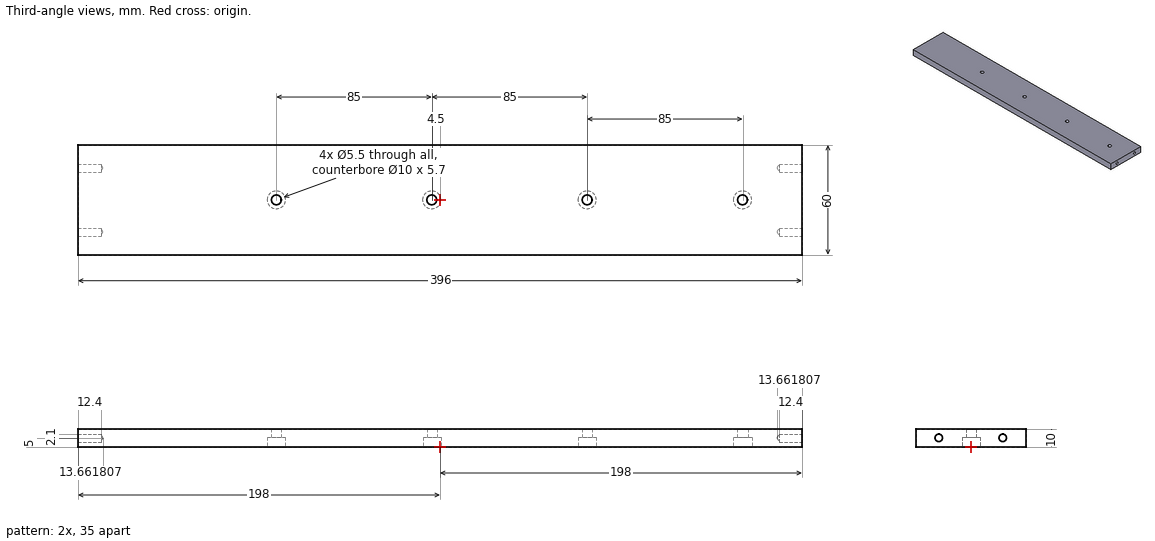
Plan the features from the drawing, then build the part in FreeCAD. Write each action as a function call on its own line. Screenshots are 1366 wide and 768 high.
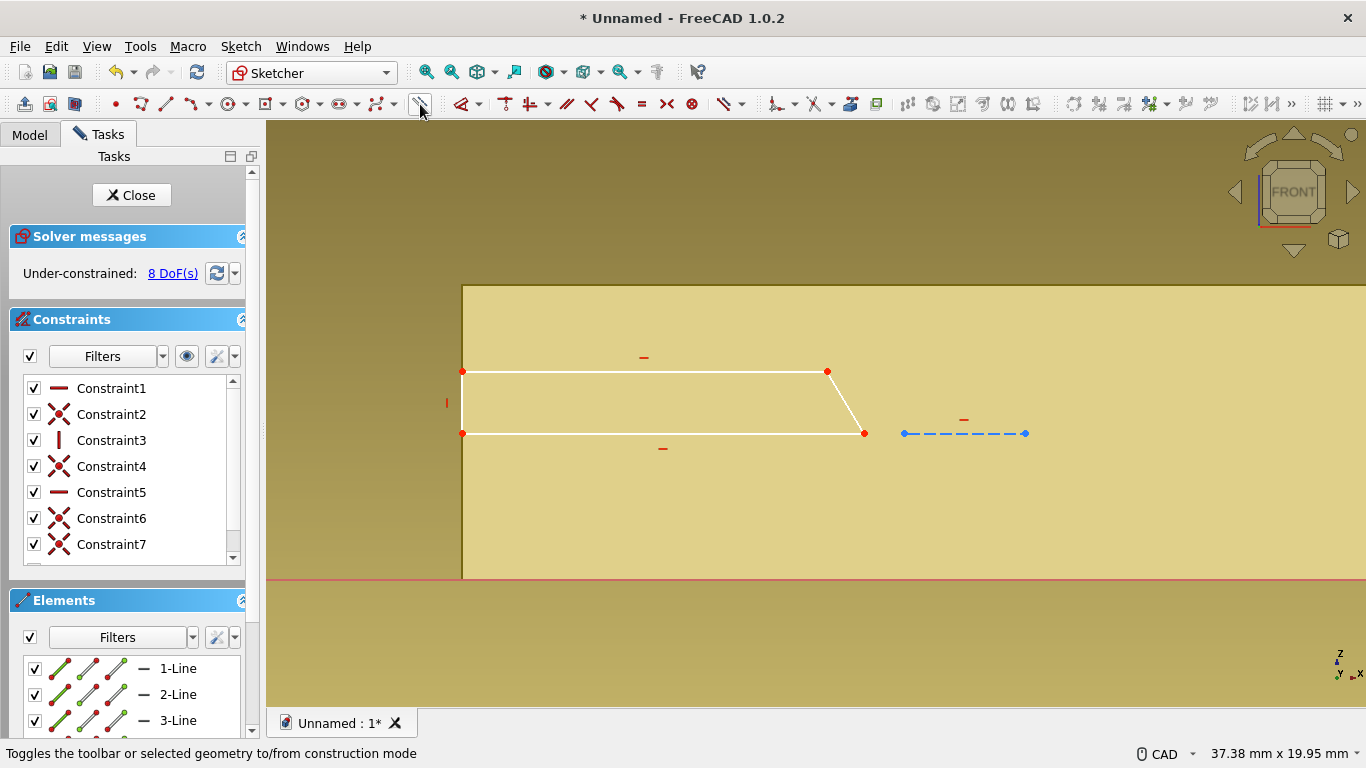
click(460, 104)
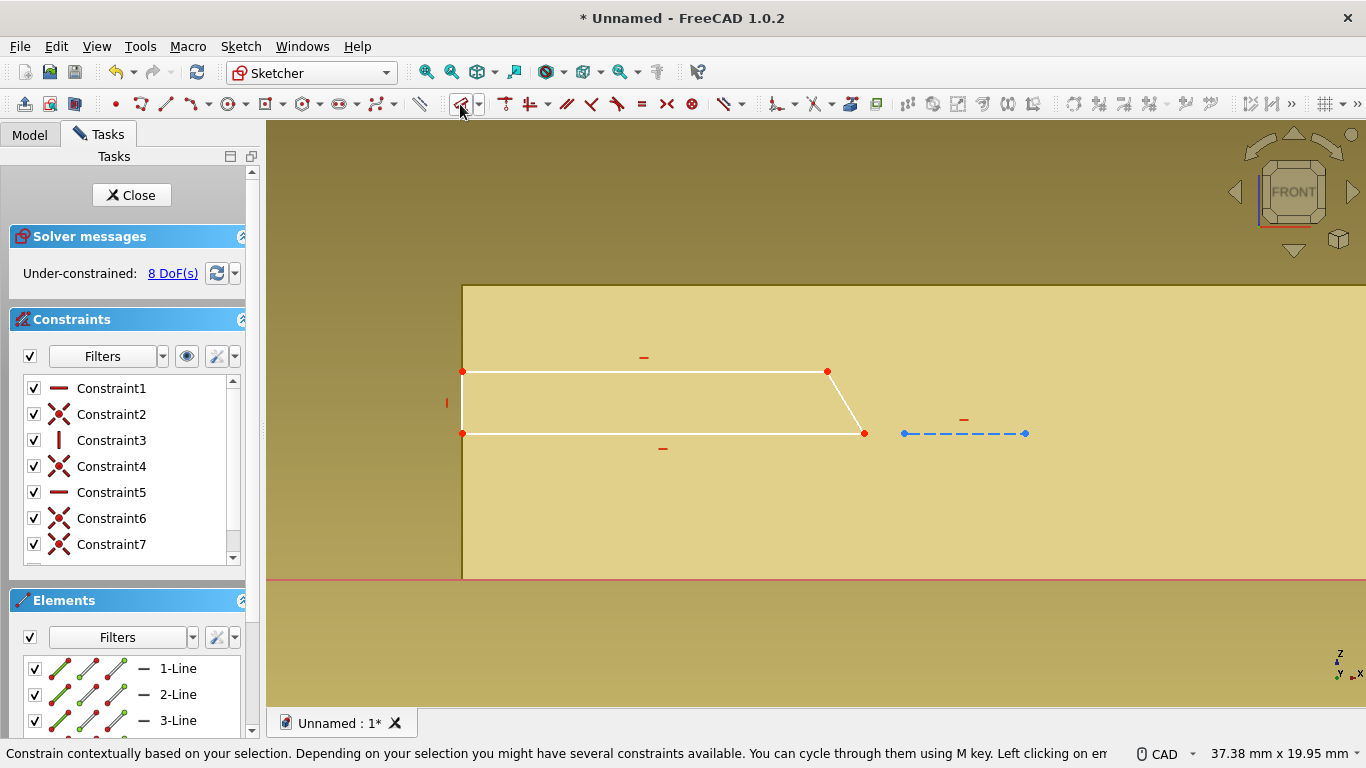
click(864, 434)
click(830, 507)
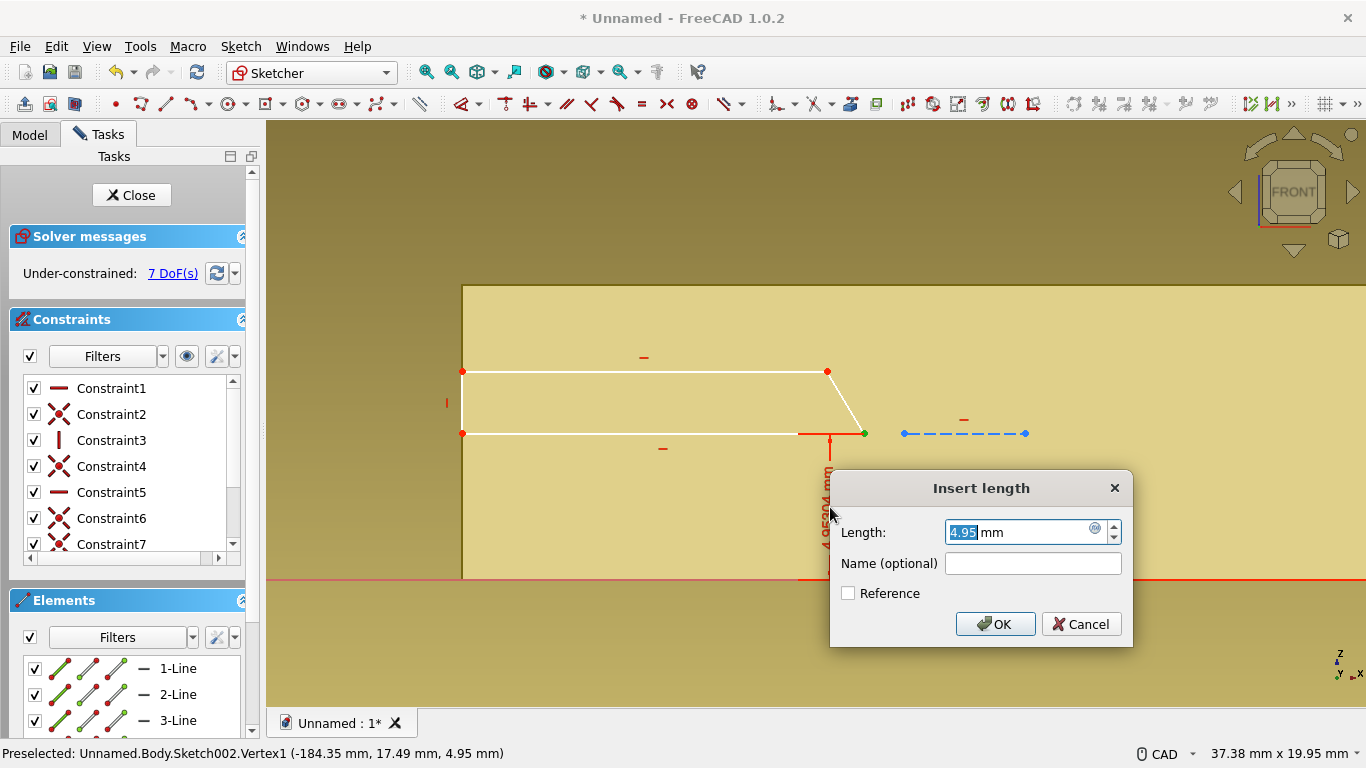
text(5)
key(Return)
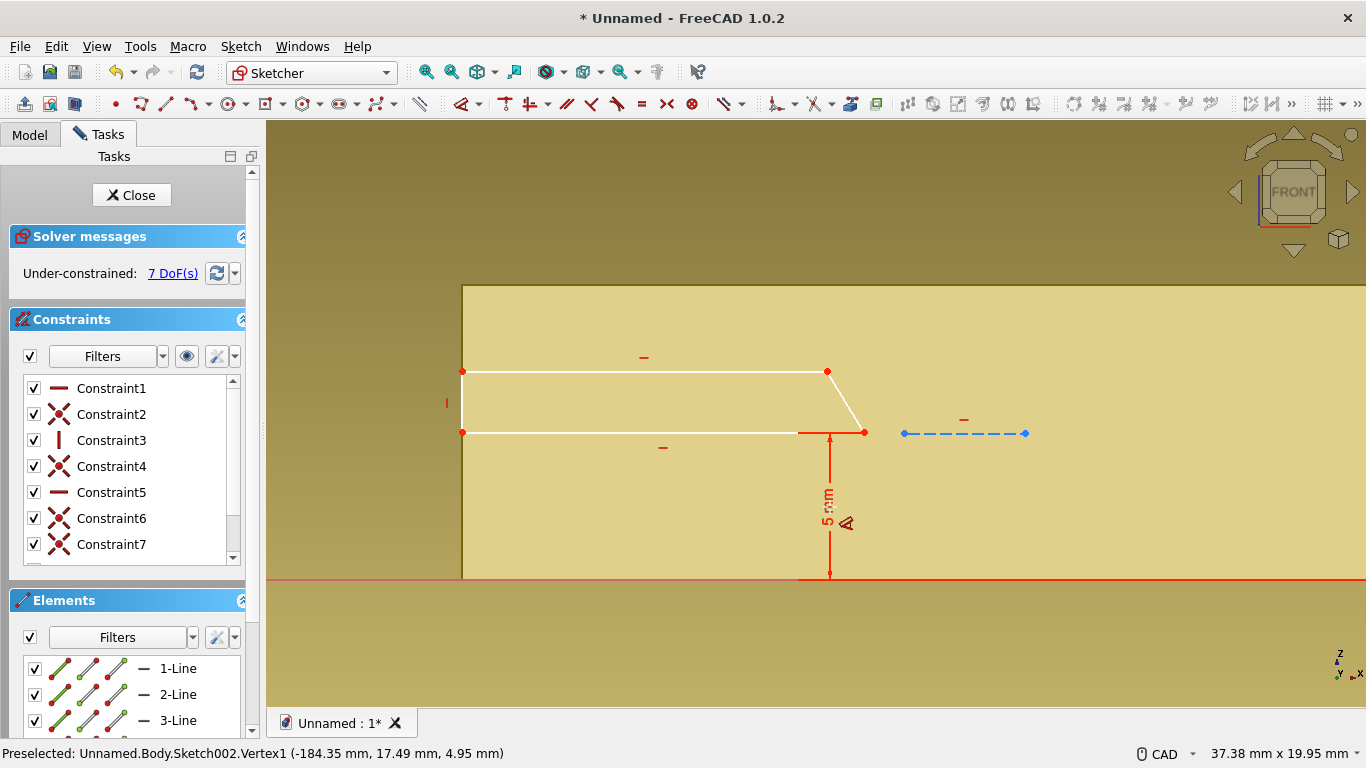
click(904, 434)
click(870, 473)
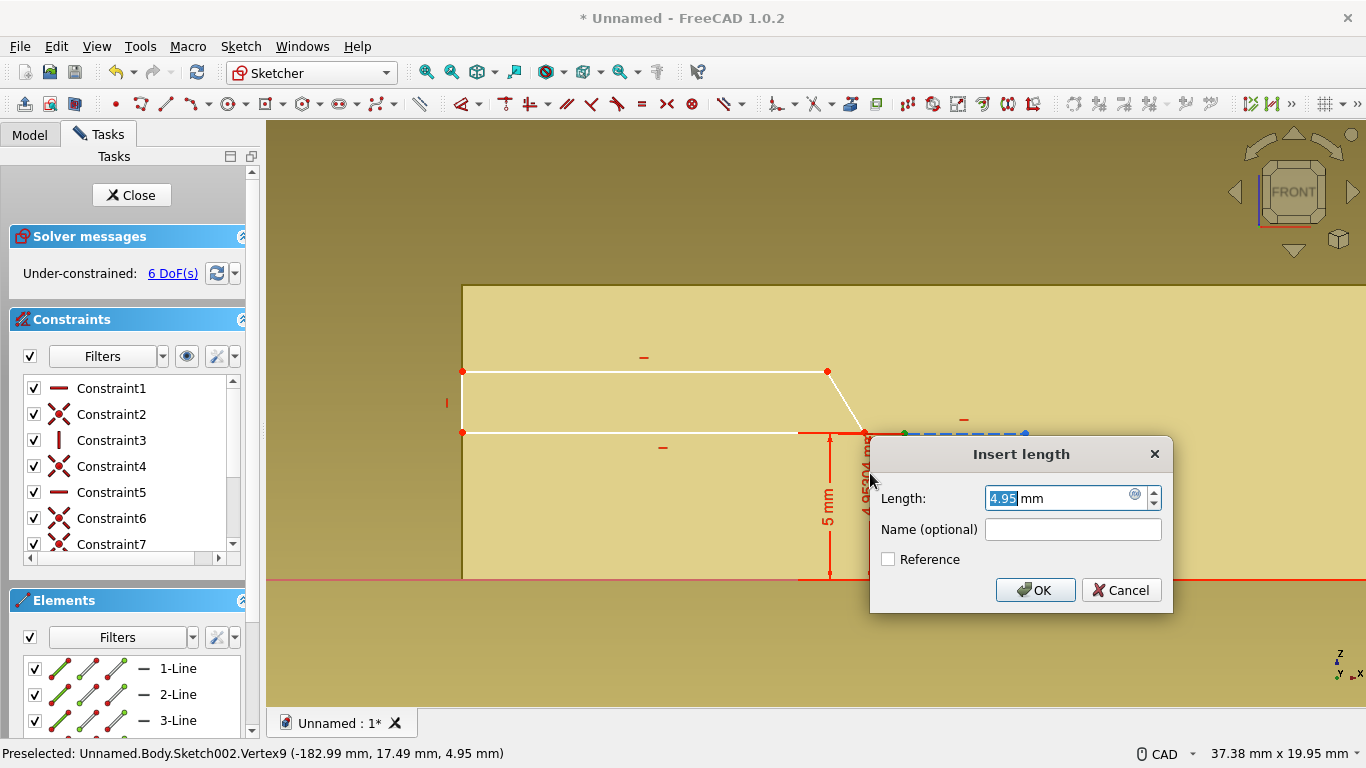
text(5)
key(Return)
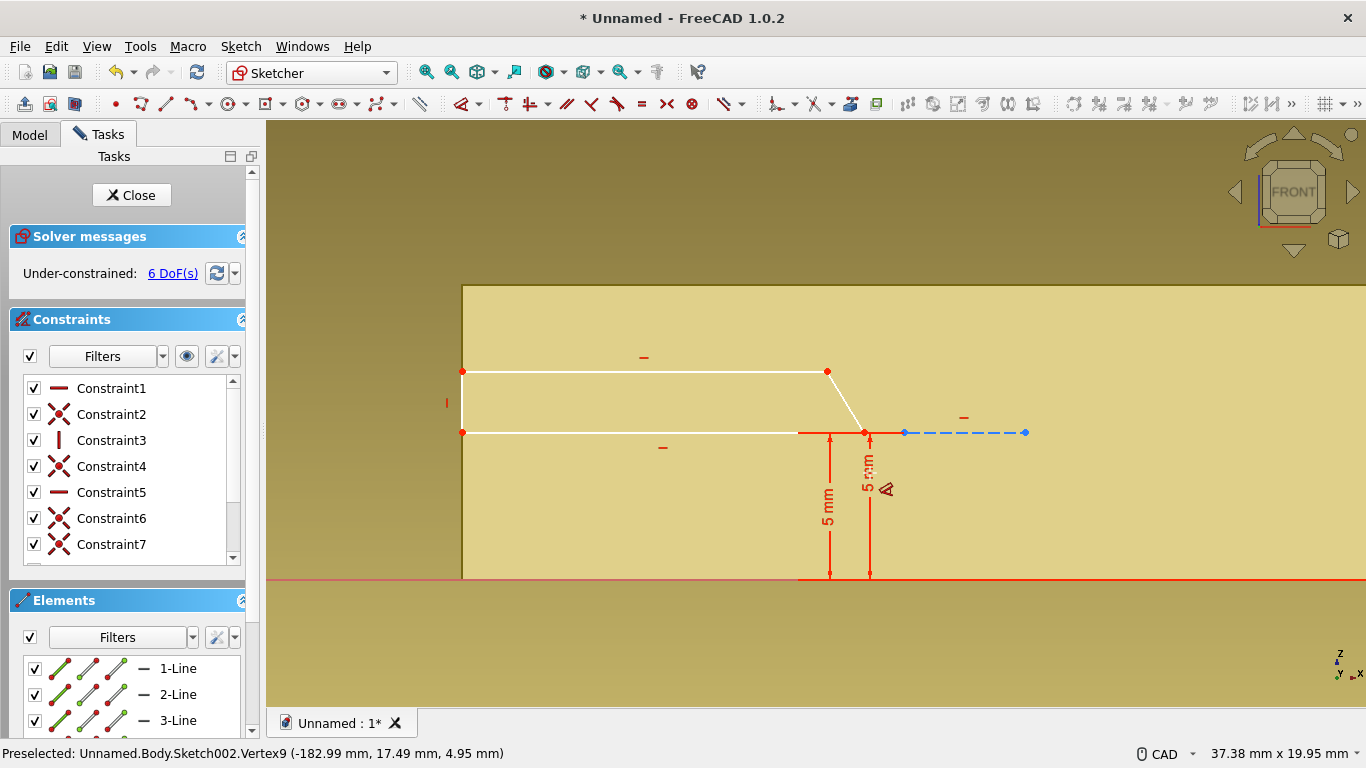
click(462, 414)
click(428, 402)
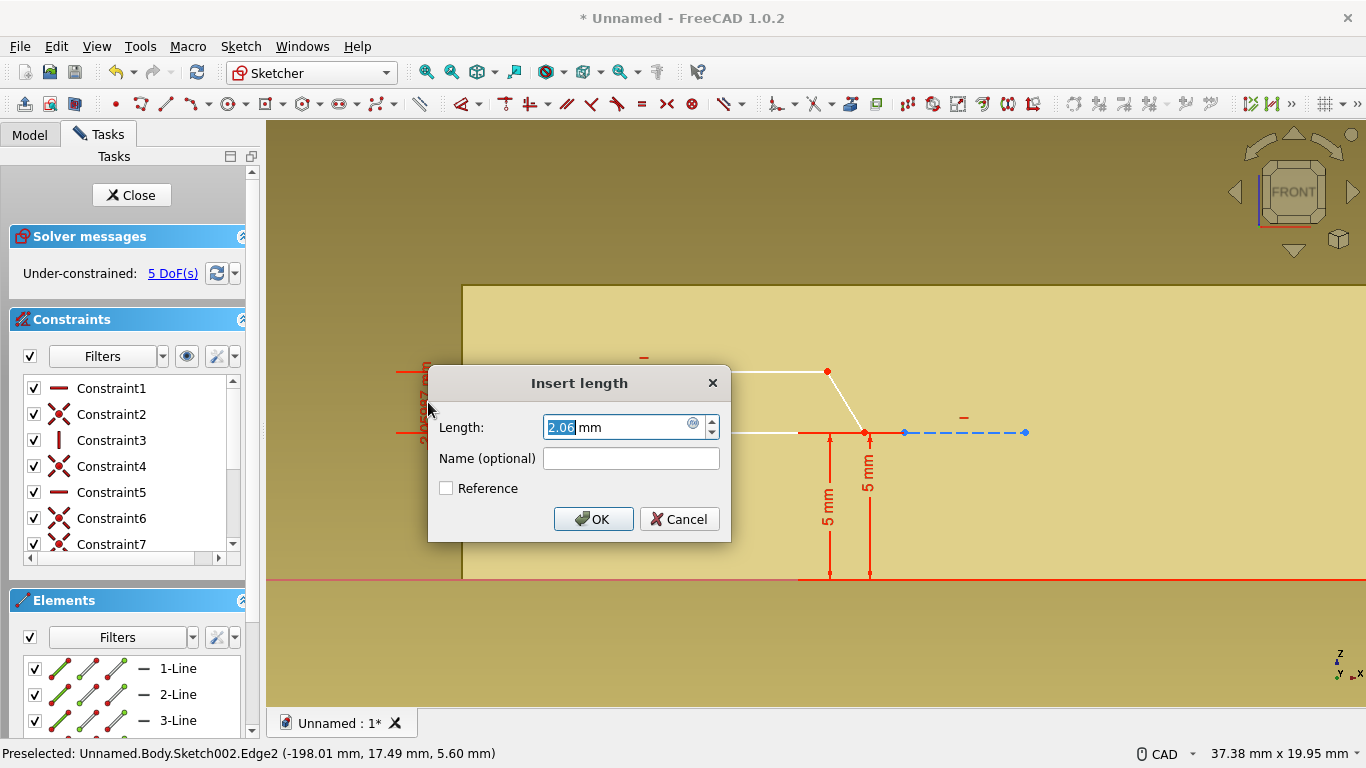
text(2.1)
key(Return)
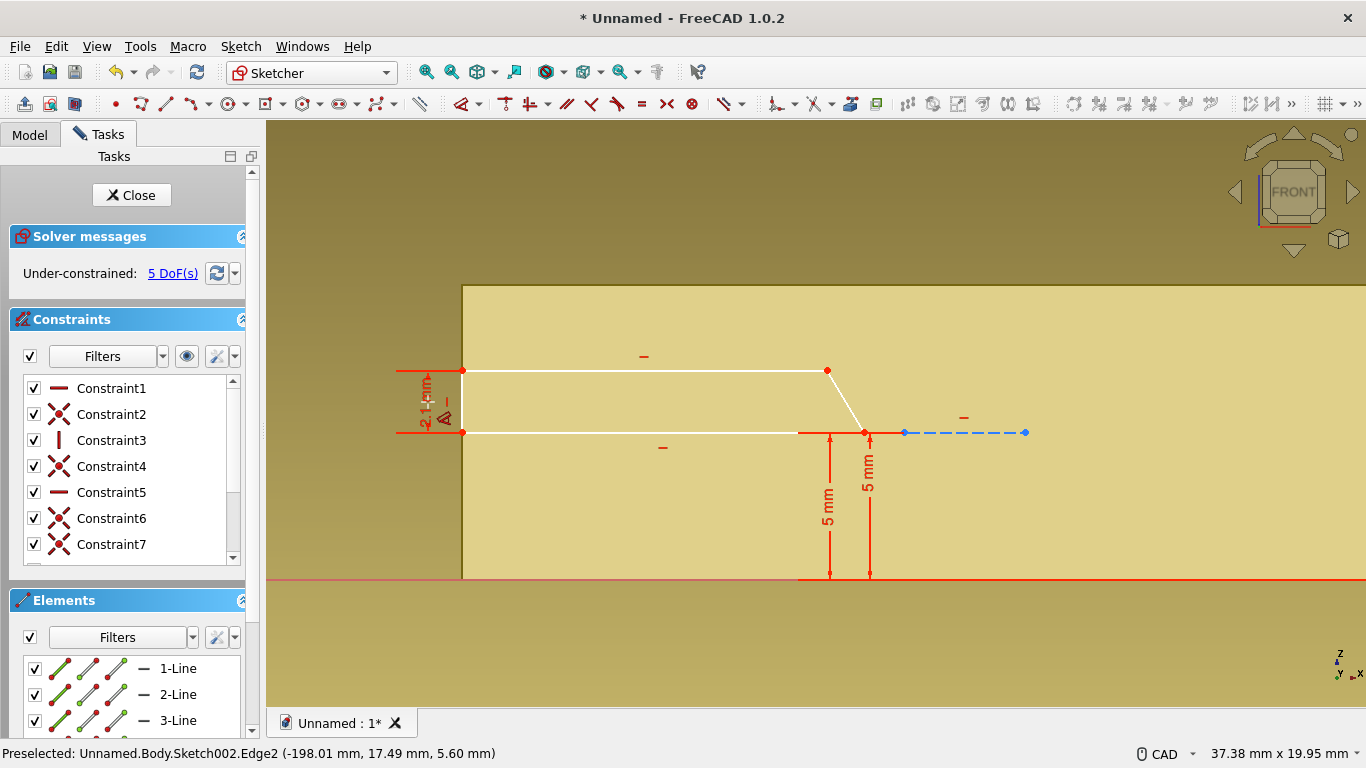
click(572, 371)
click(645, 337)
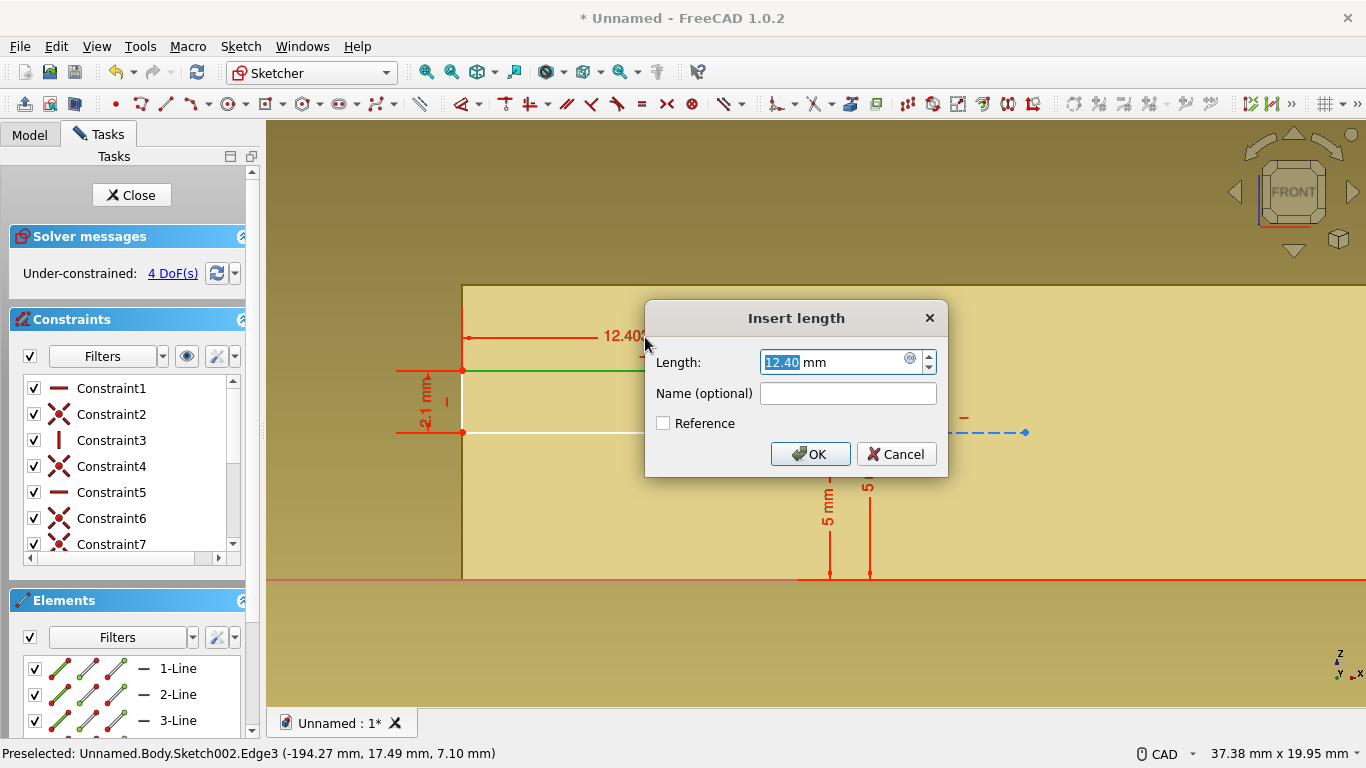
text(12.4)
key(Return)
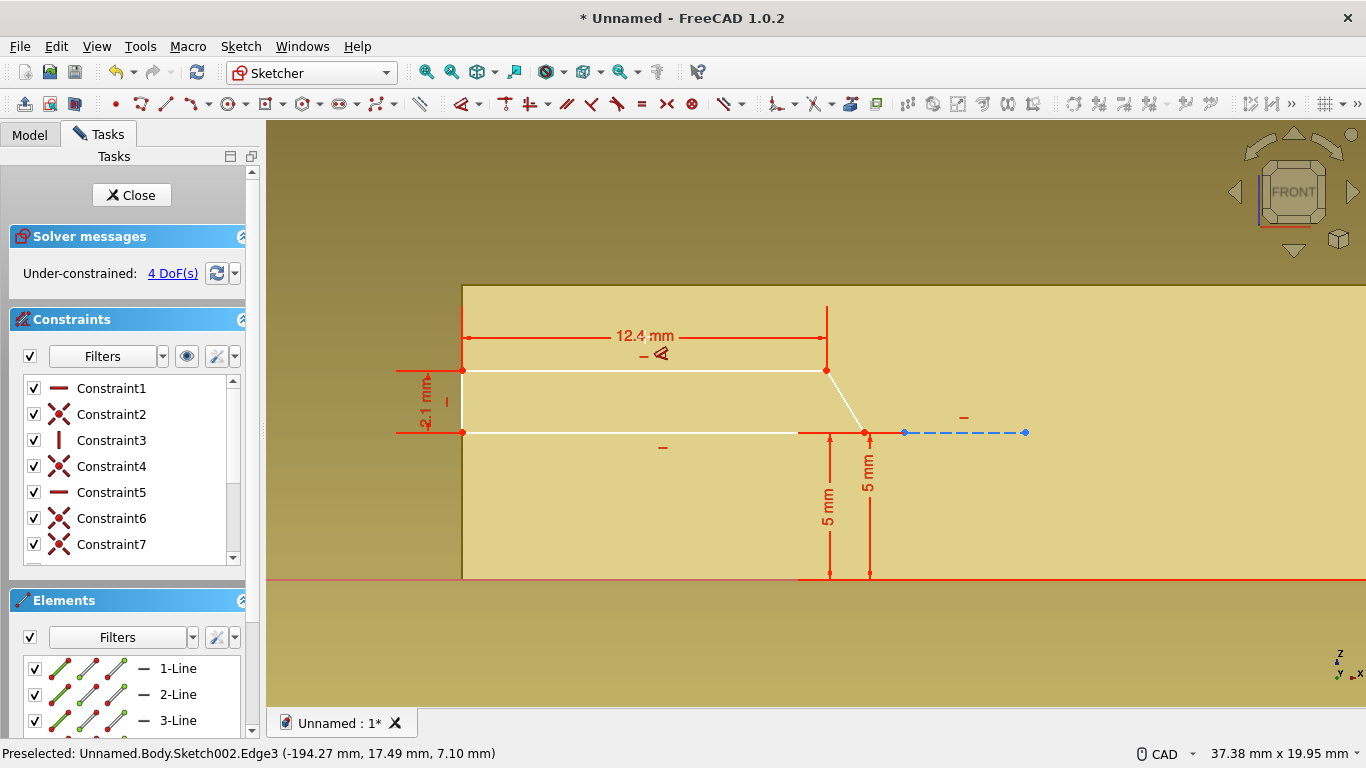
click(462, 433)
click(832, 614)